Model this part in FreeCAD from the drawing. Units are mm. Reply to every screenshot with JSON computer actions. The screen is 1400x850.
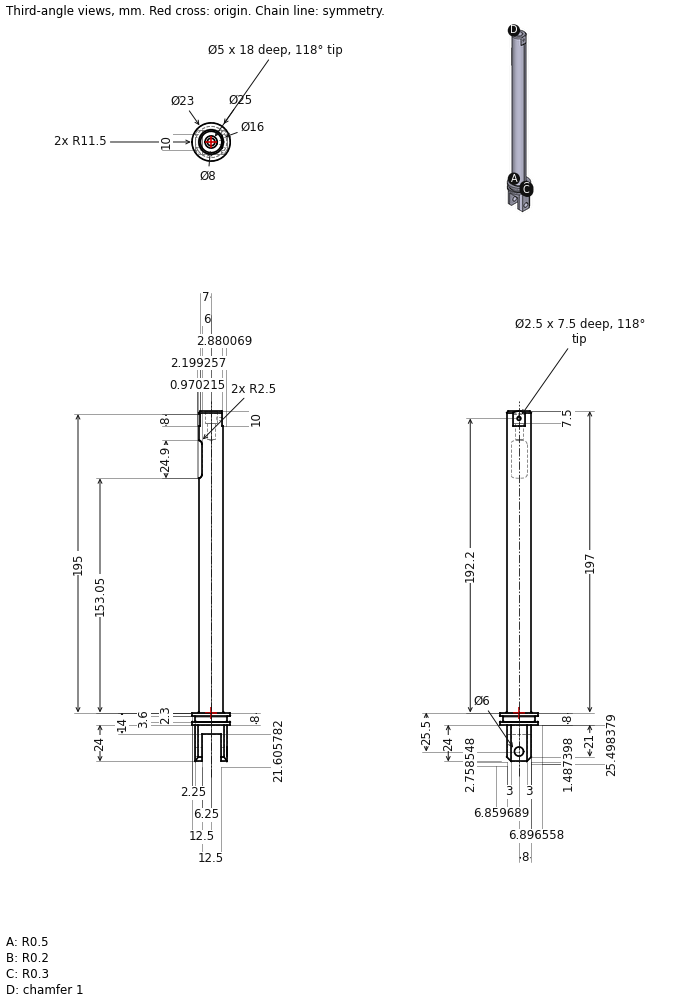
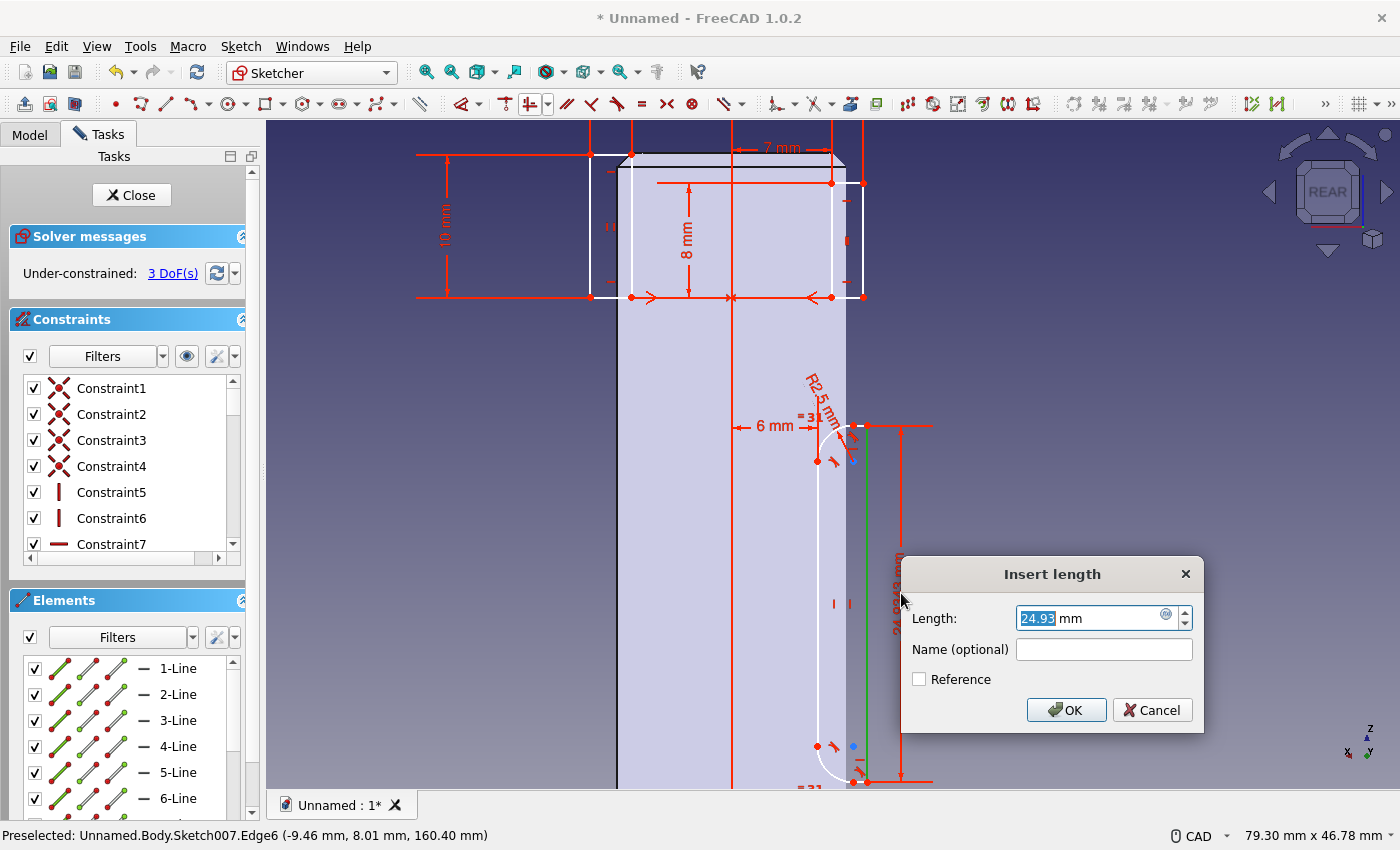
{"action": "type", "text": "24.9"}
{"action": "key", "text": "Return"}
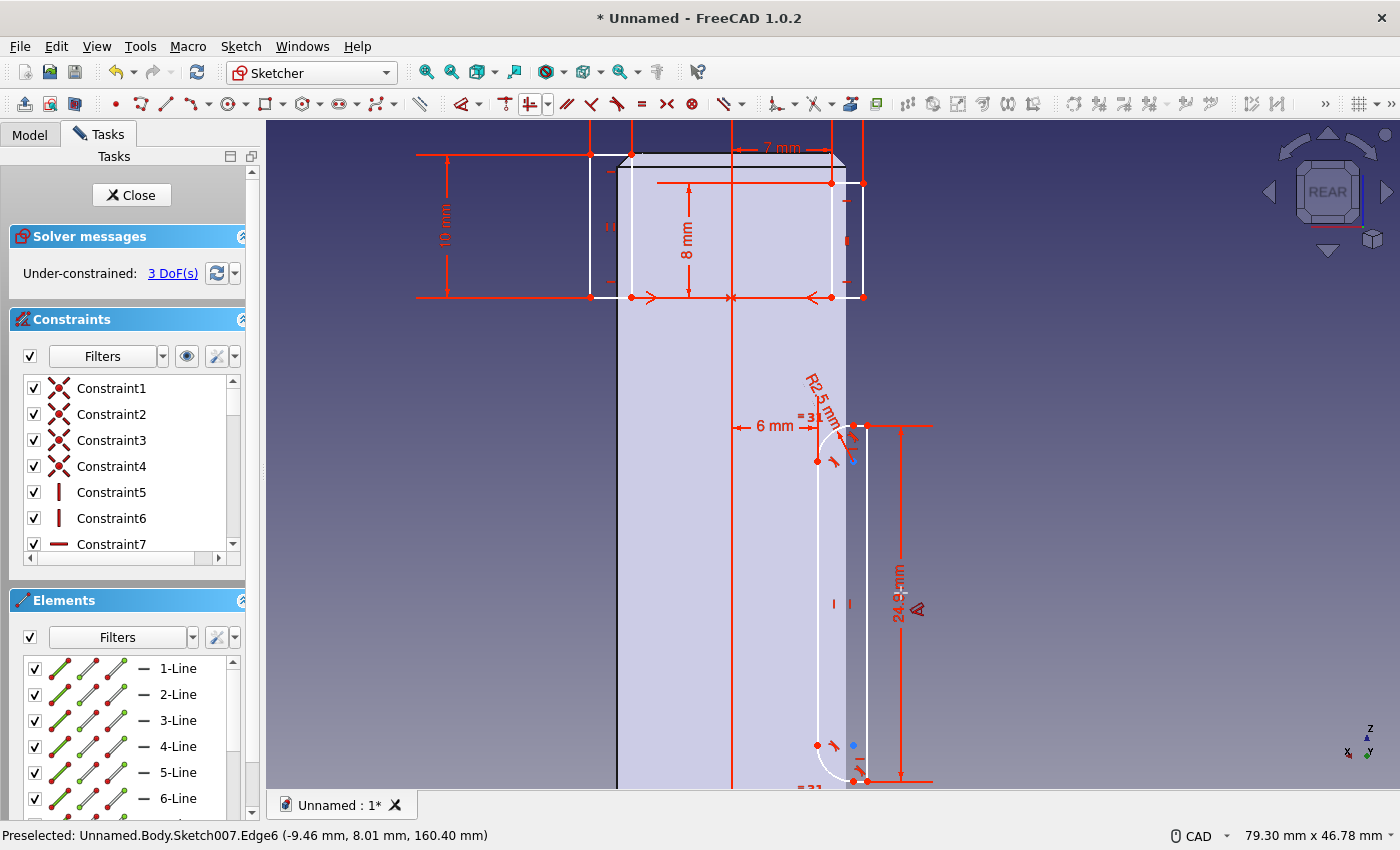
{"action": "left_click", "coordinate": [832, 183]}
{"action": "left_click", "coordinate": [866, 339]}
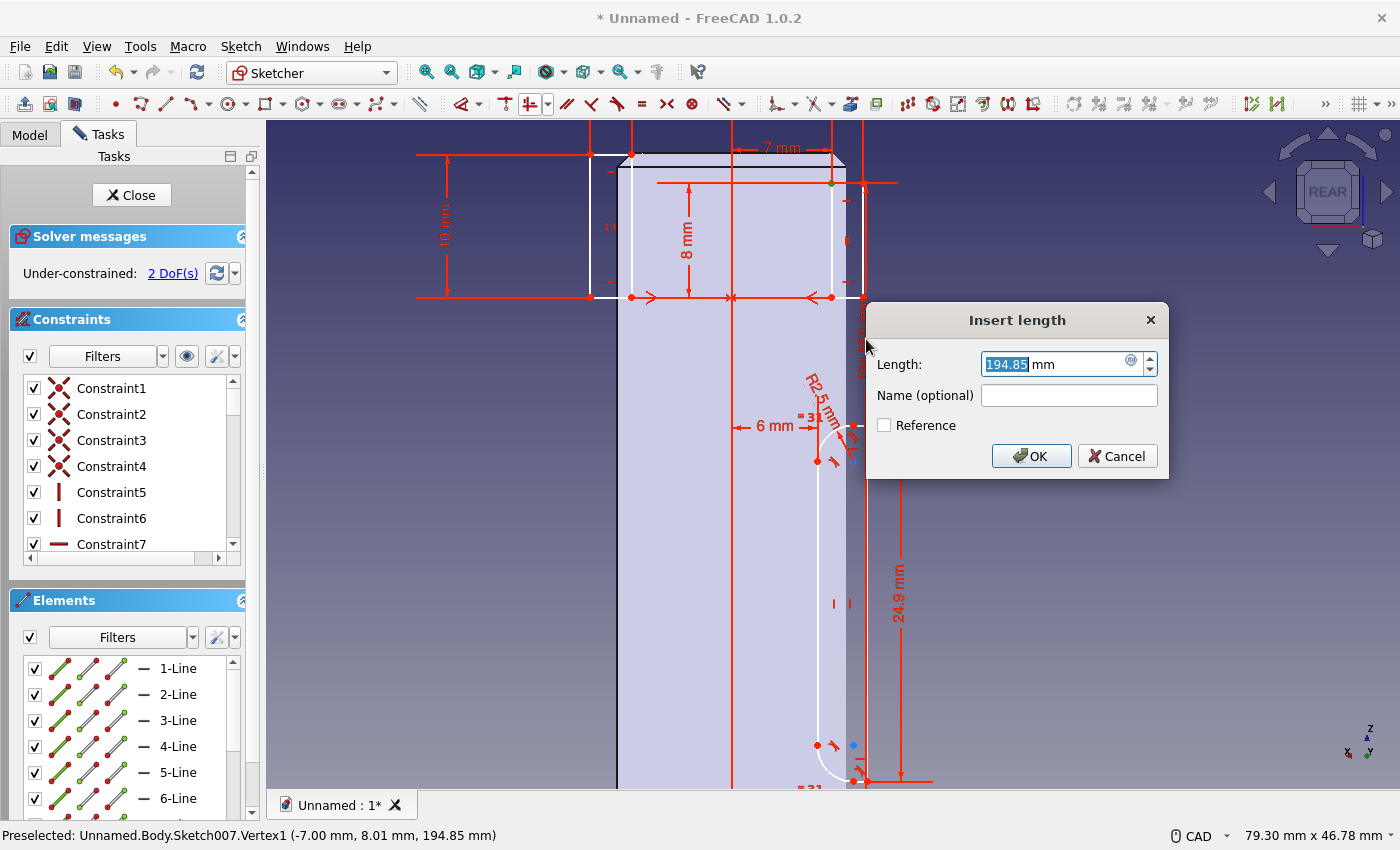
{"action": "type", "text": "195"}
{"action": "key", "text": "Return"}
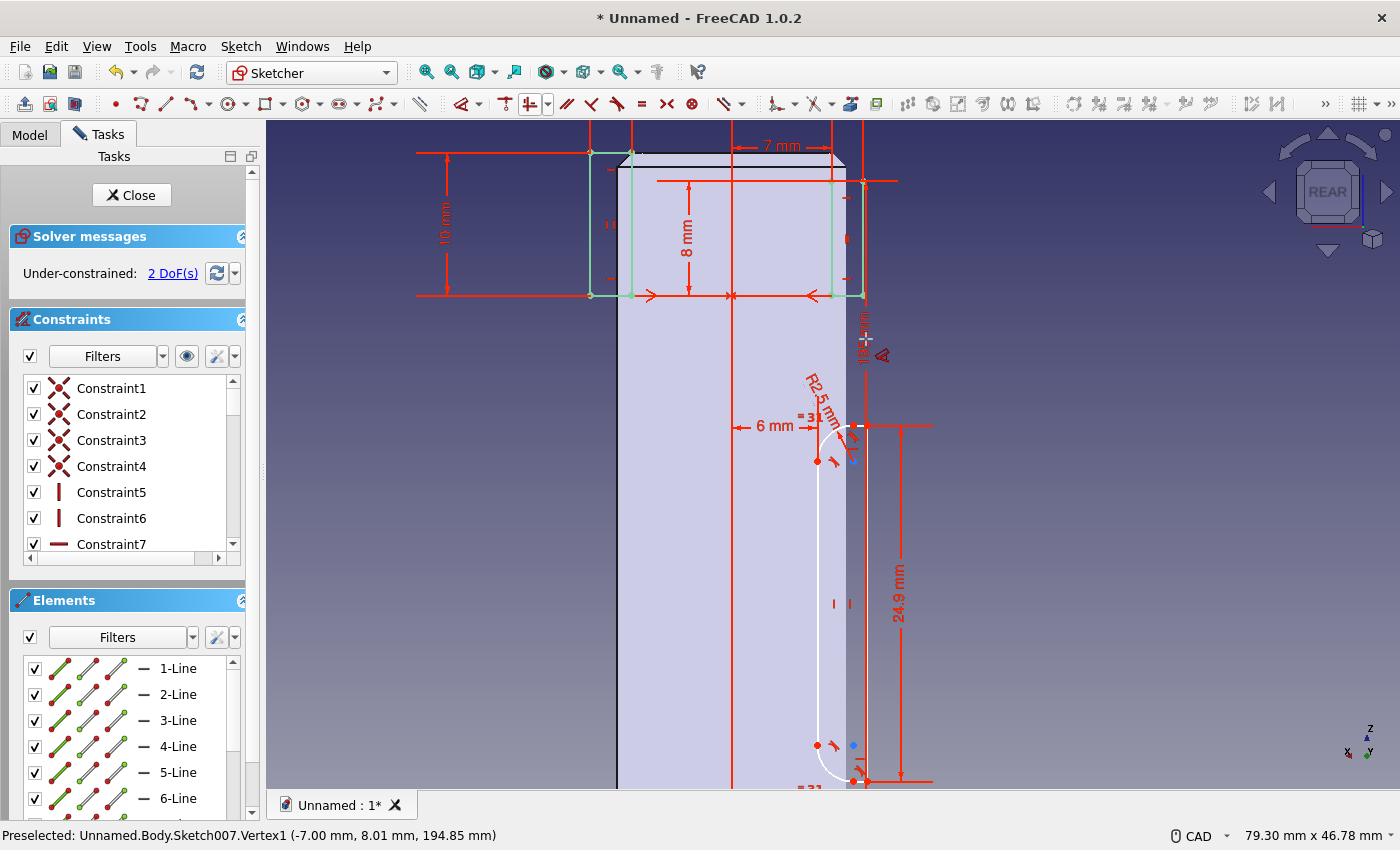
{"action": "scroll", "coordinate": [837, 429], "scroll_direction": "down", "scroll_amount": 2}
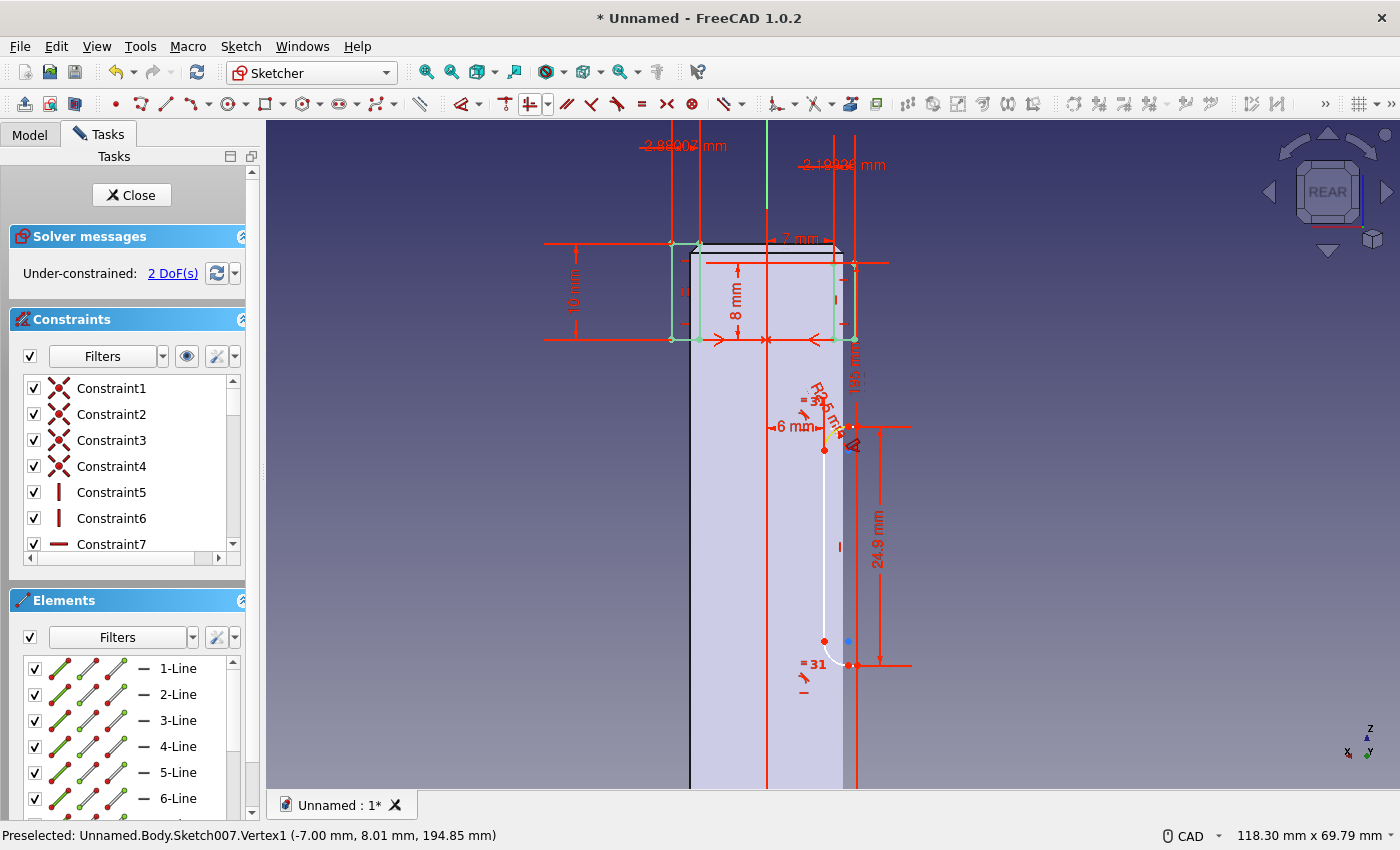
{"action": "scroll", "coordinate": [848, 666], "scroll_direction": "up", "scroll_amount": 2}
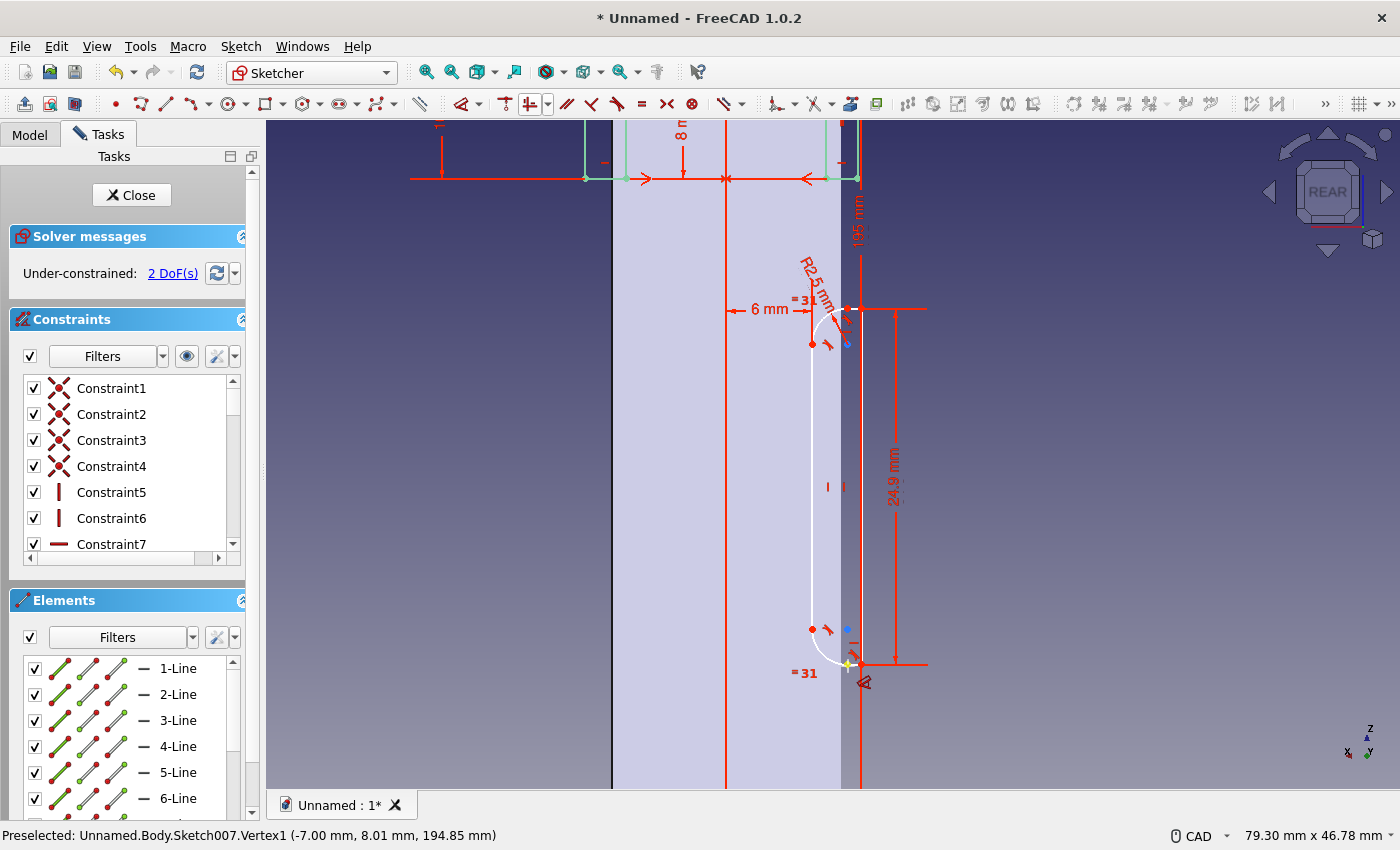
{"action": "left_click", "coordinate": [848, 665]}
{"action": "left_click", "coordinate": [882, 713]}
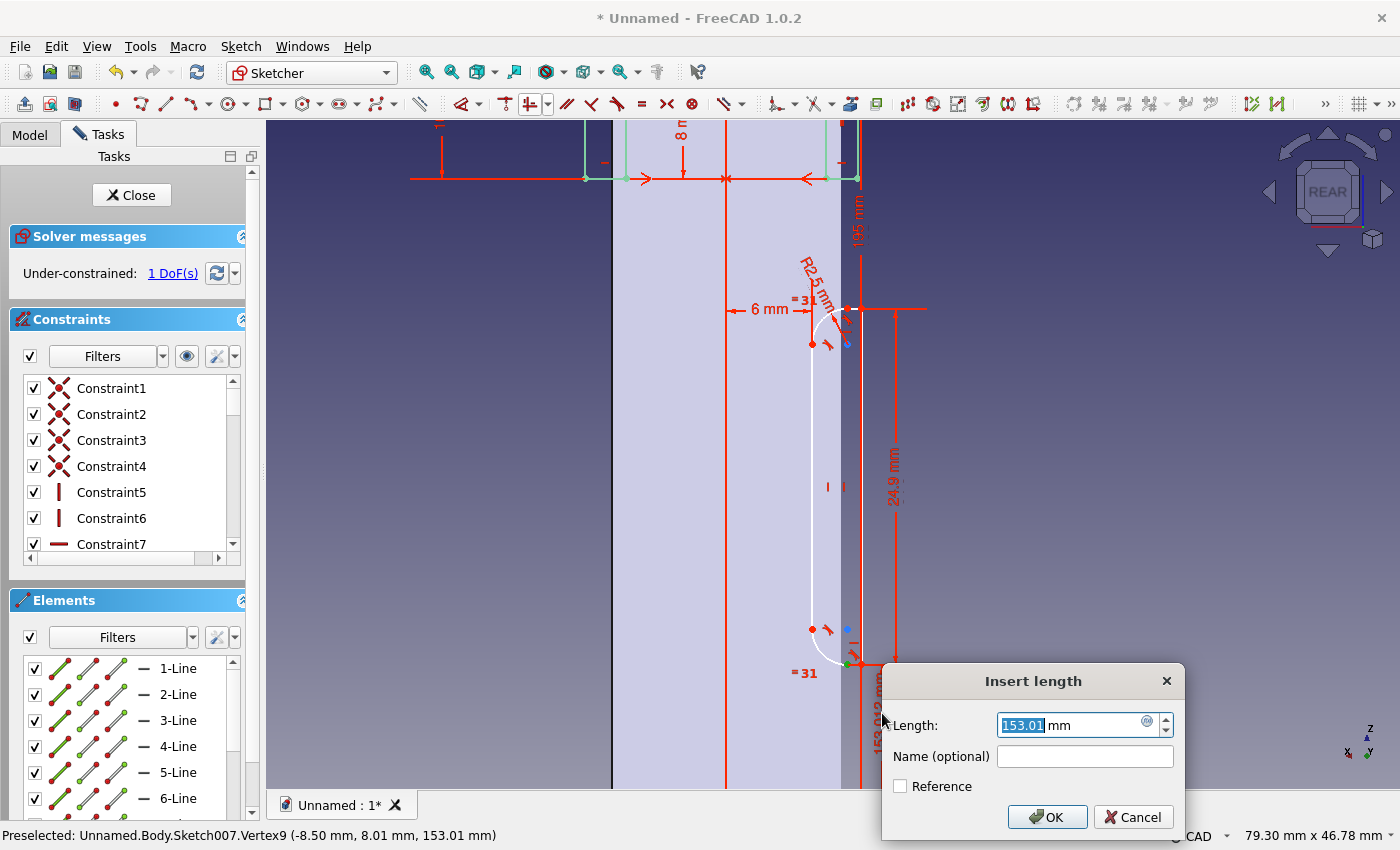
{"action": "type", "text": "153.05"}
{"action": "key", "text": "Return"}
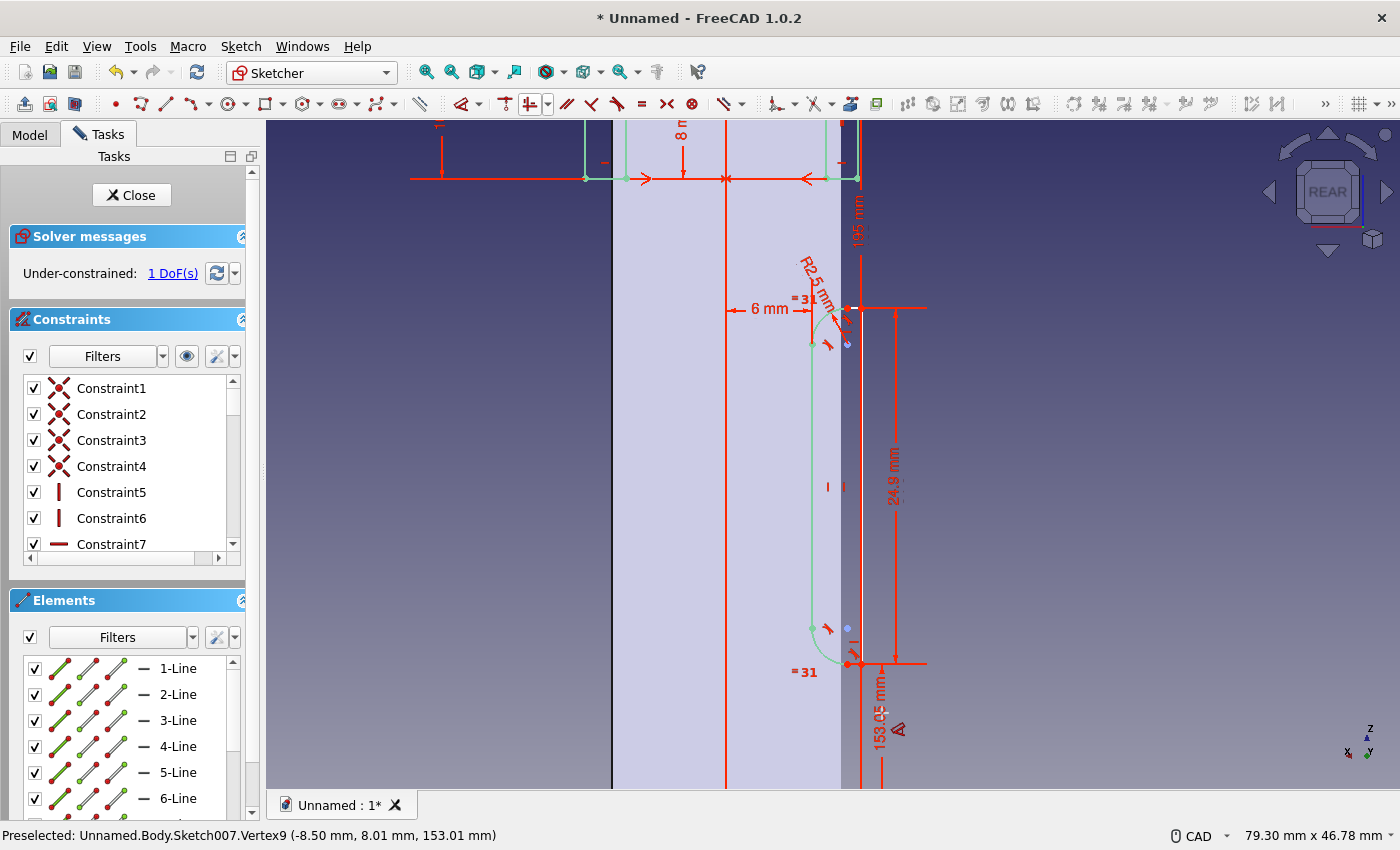
{"action": "scroll", "coordinate": [855, 664], "scroll_direction": "up", "scroll_amount": 6}